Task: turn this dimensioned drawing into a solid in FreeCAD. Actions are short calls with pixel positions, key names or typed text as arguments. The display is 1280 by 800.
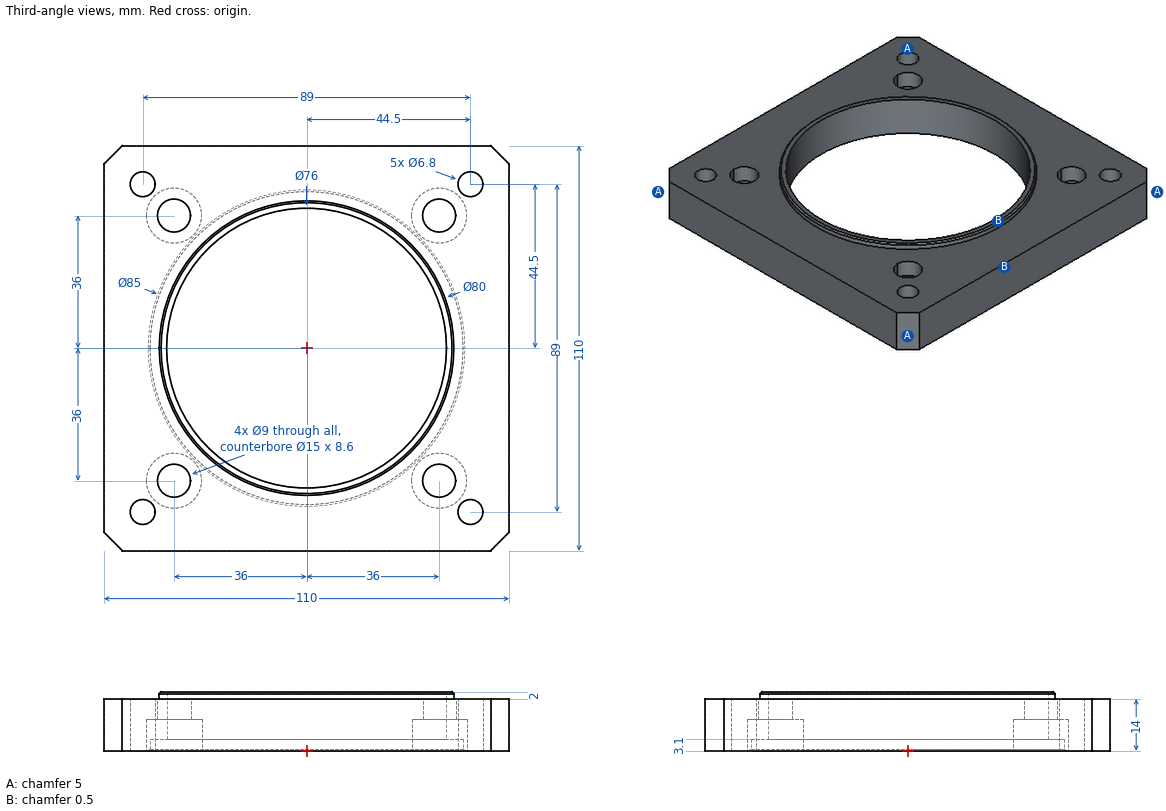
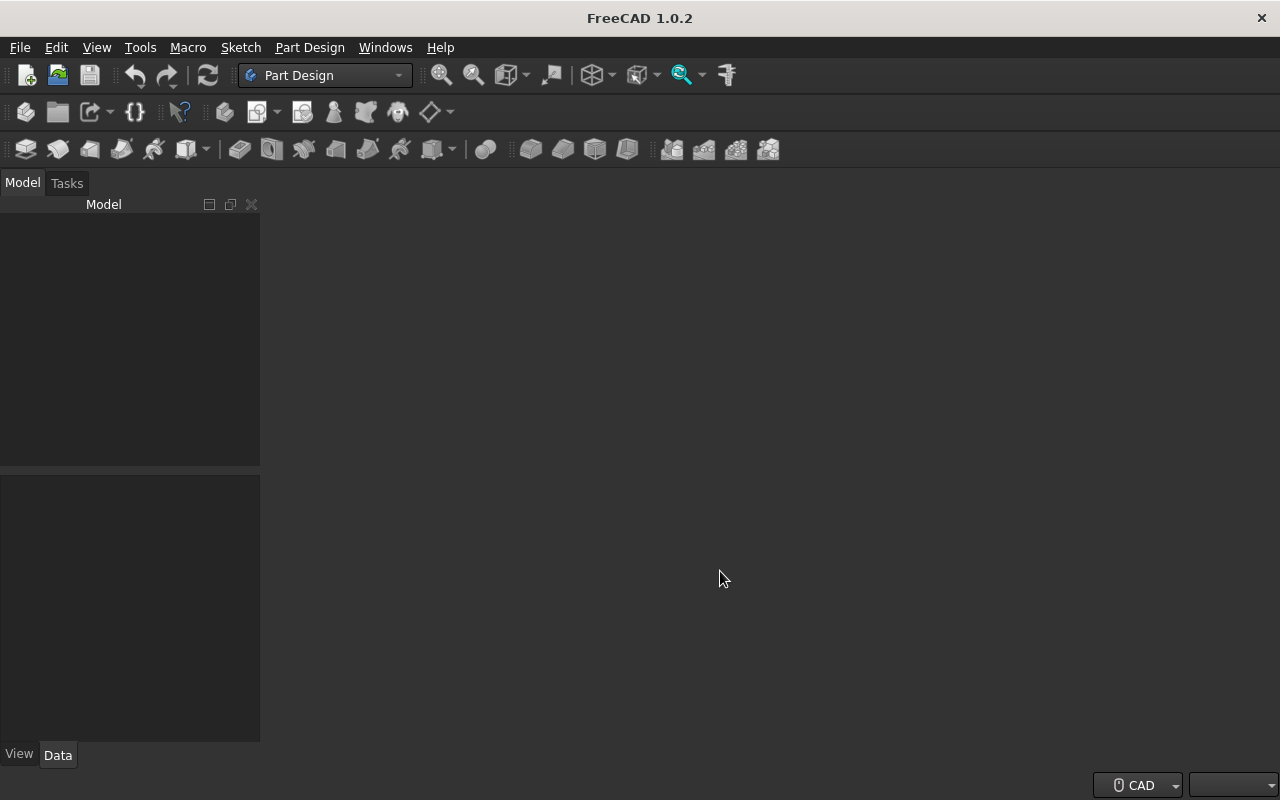
click(26, 76)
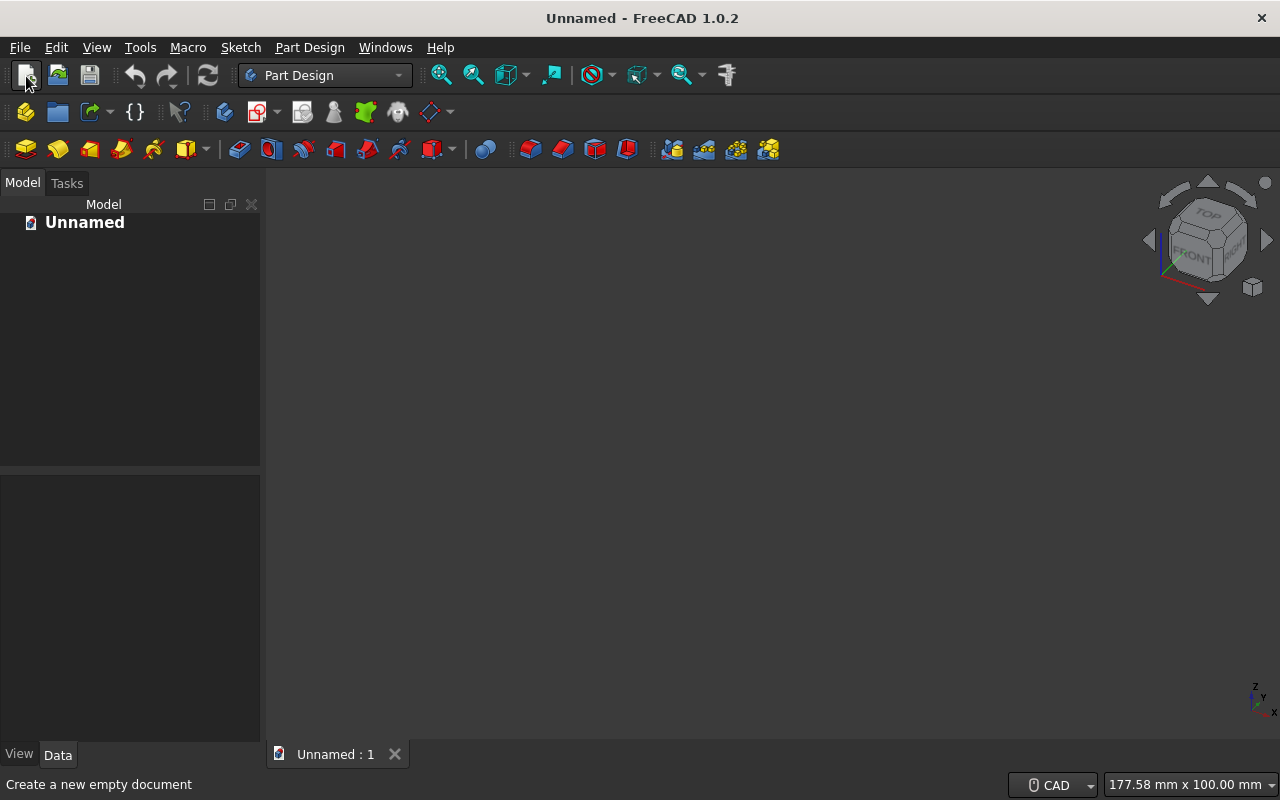
click(258, 112)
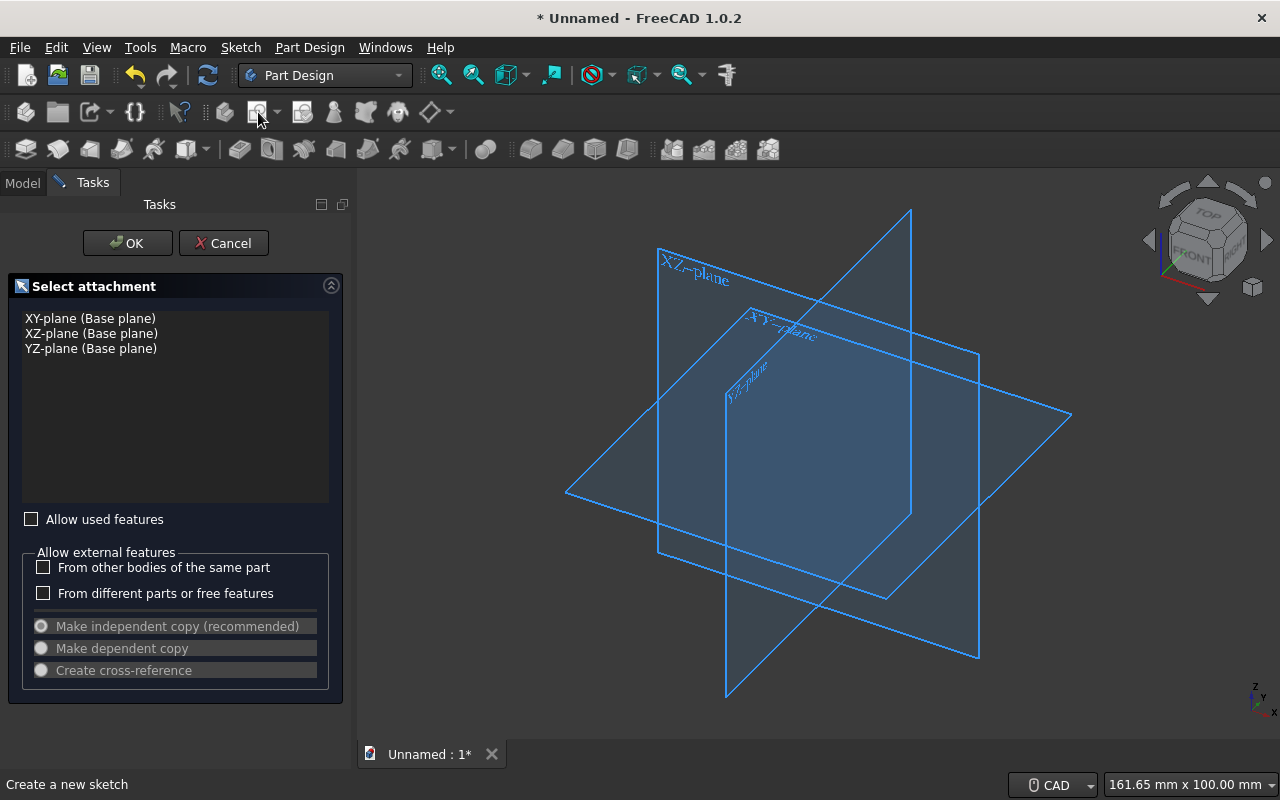
click(82, 318)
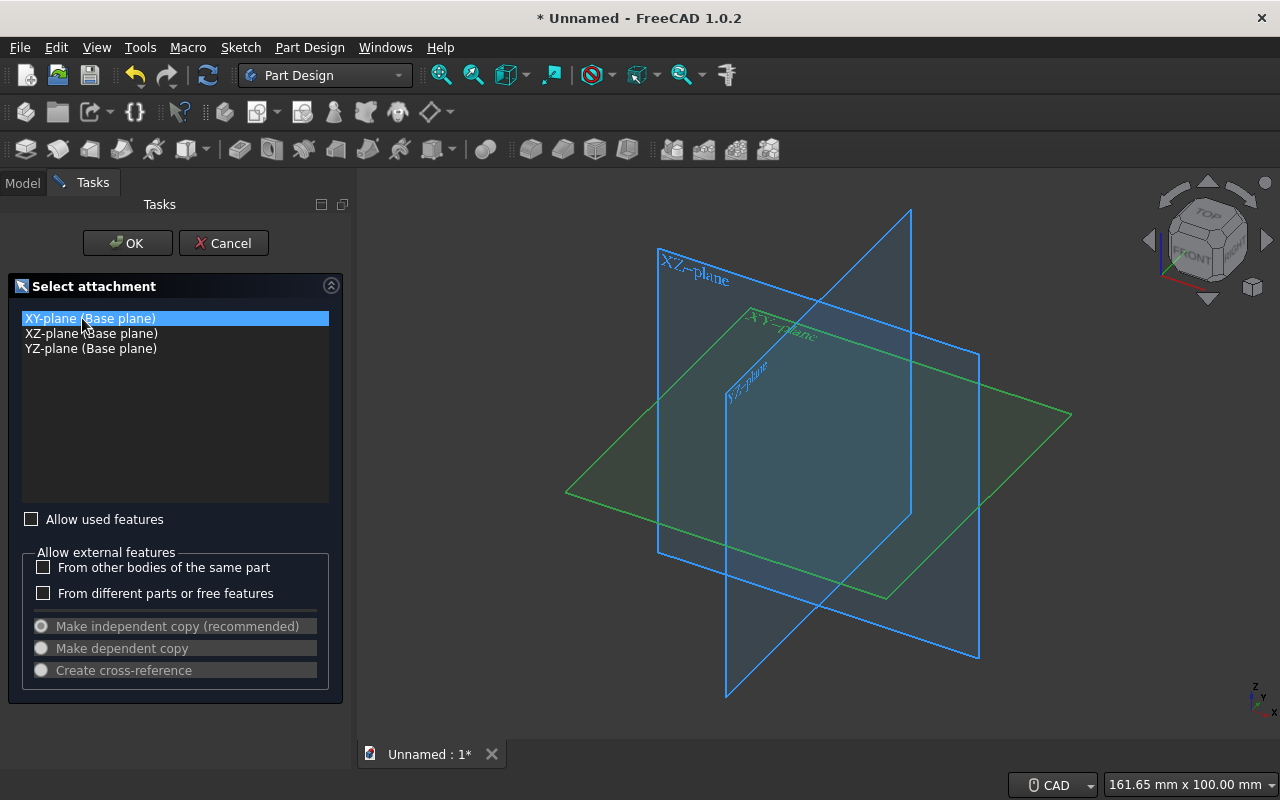
click(128, 243)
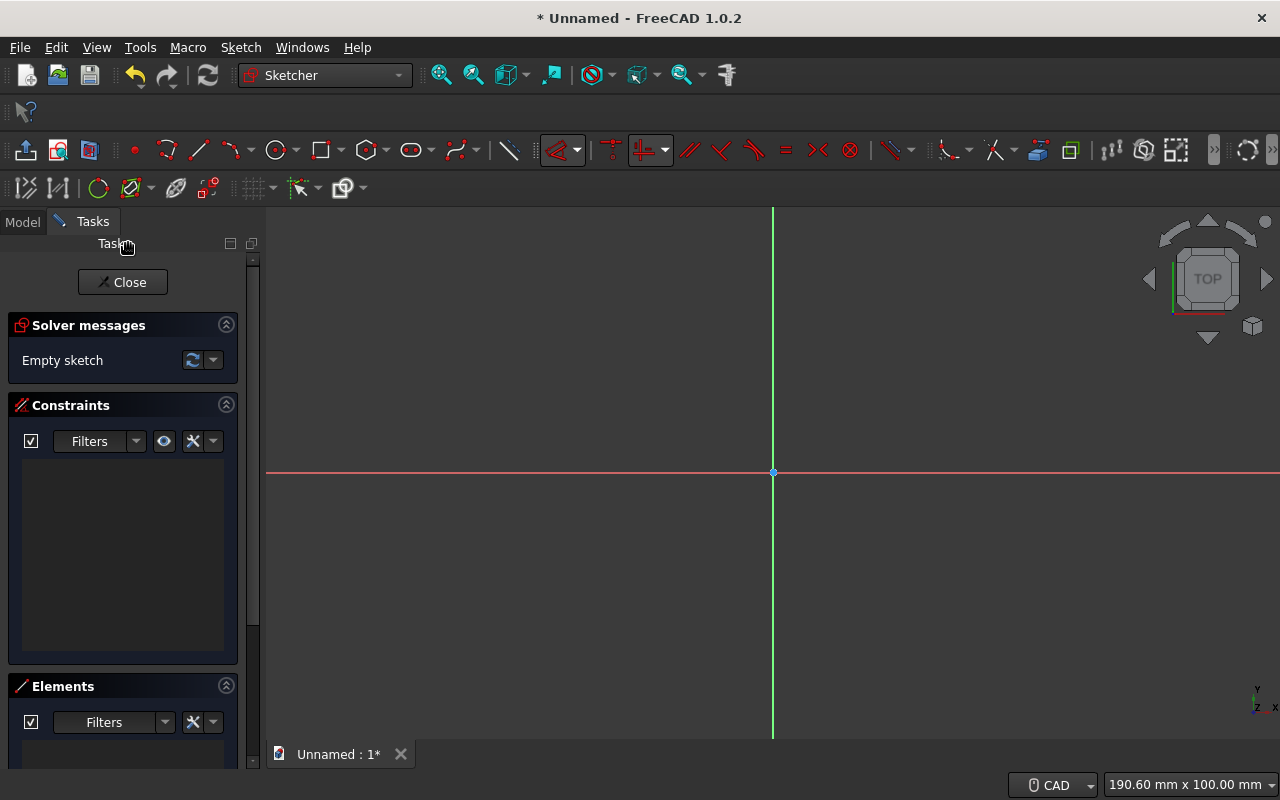
scroll(621, 473, down, 3)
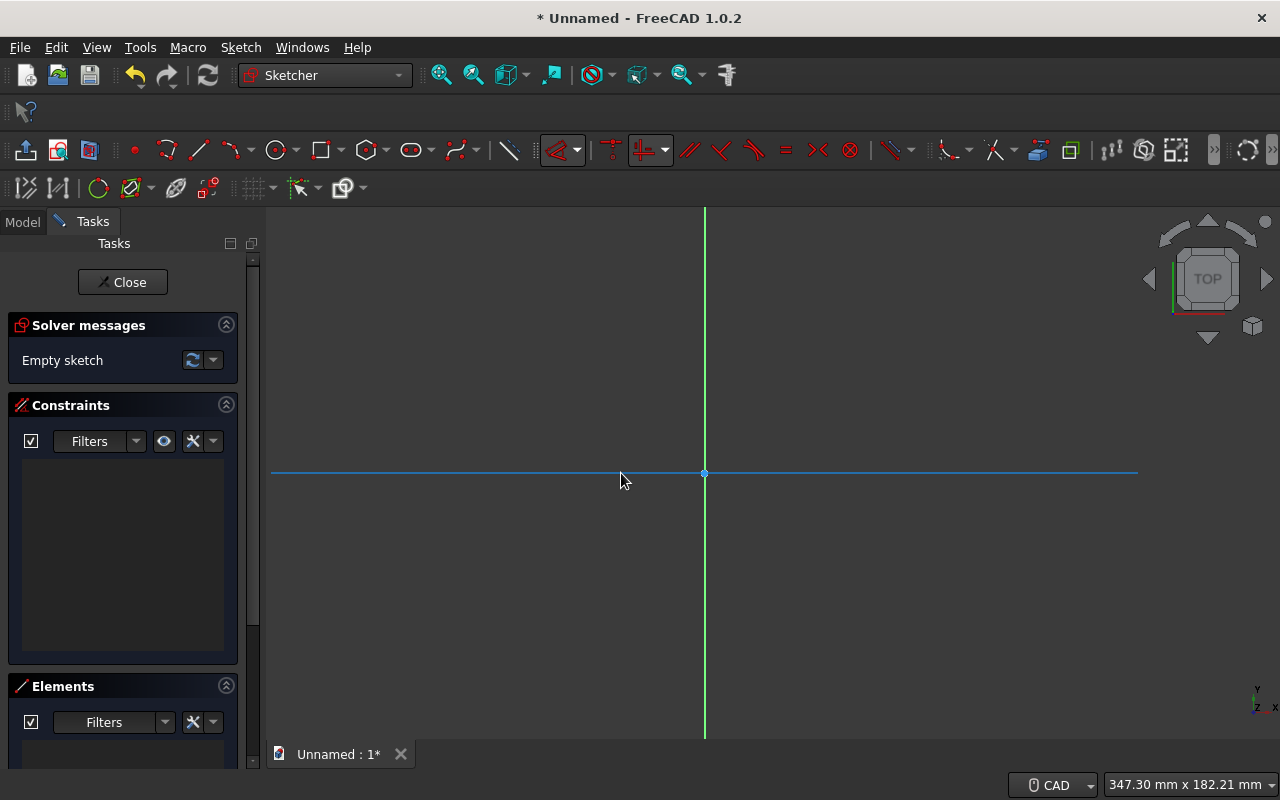
key(g)
key(v)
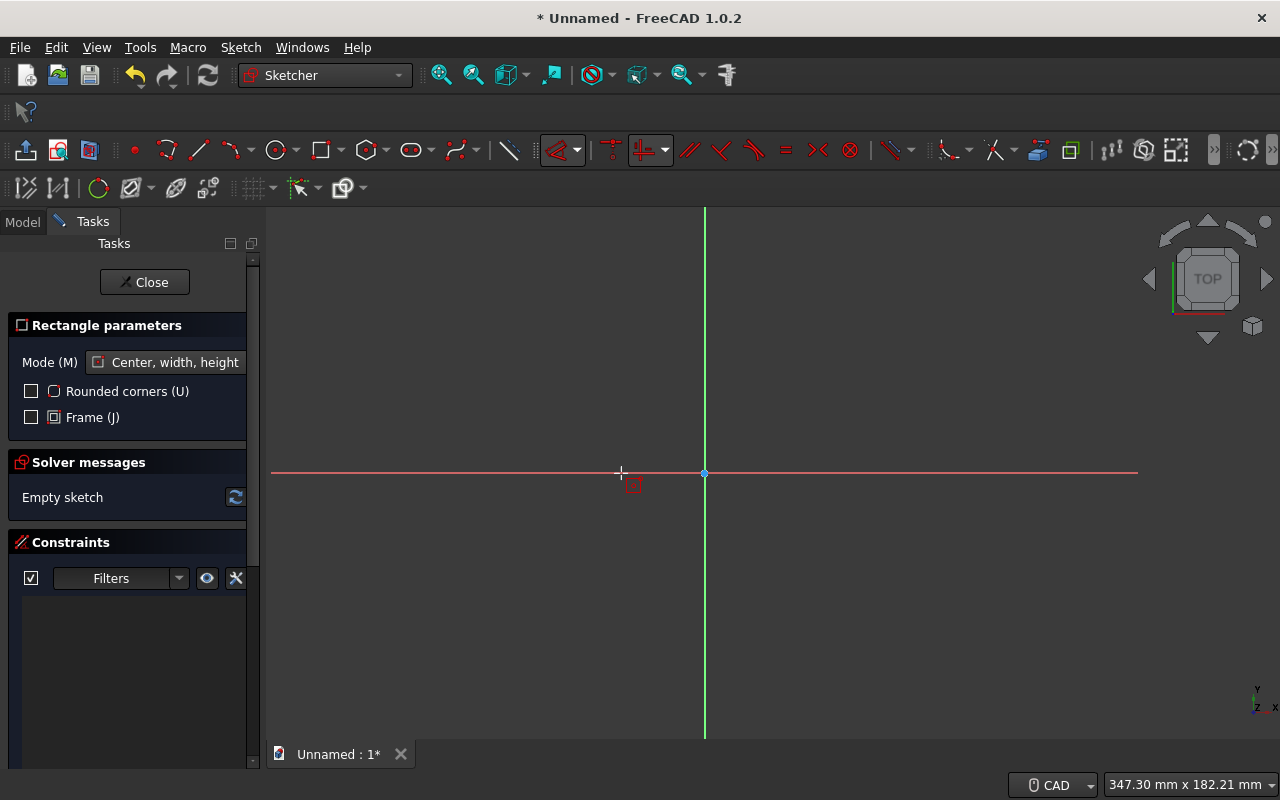
click(705, 473)
click(865, 313)
key(Escape)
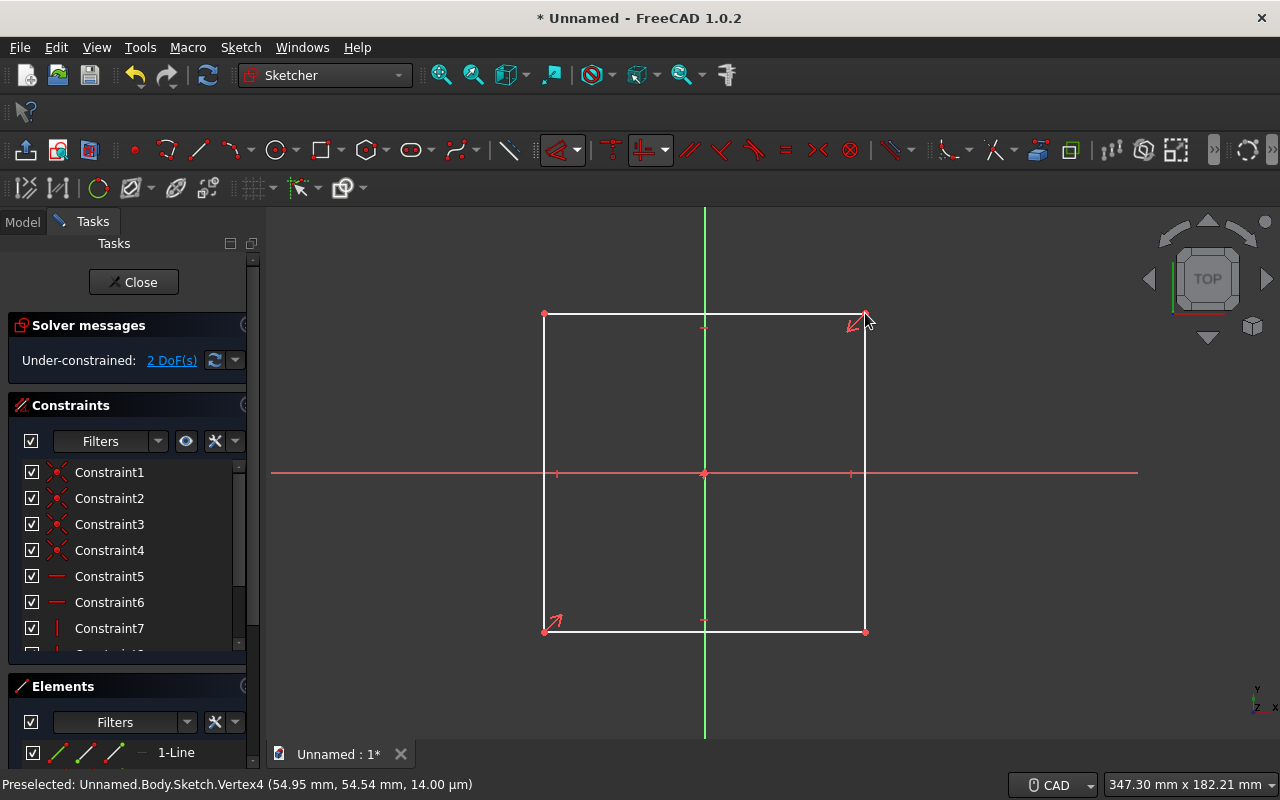
click(640, 632)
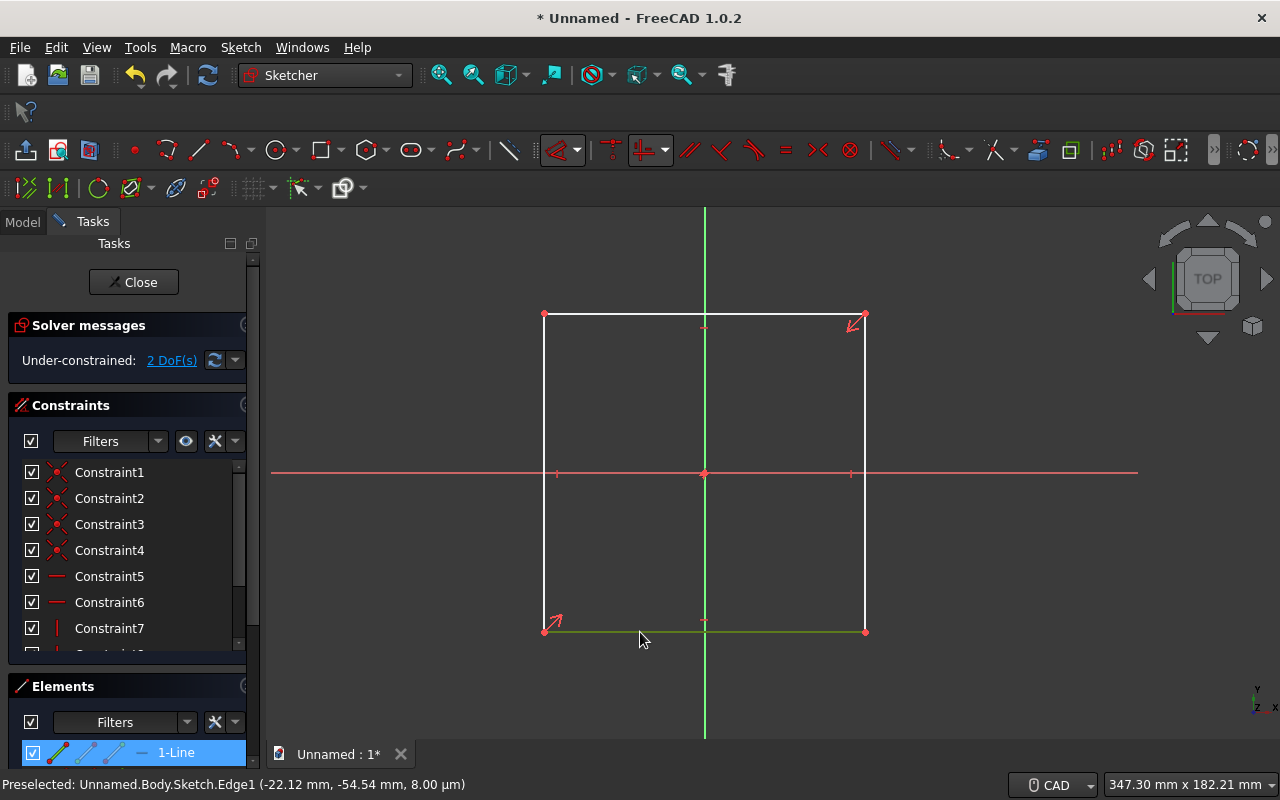
click(580, 150)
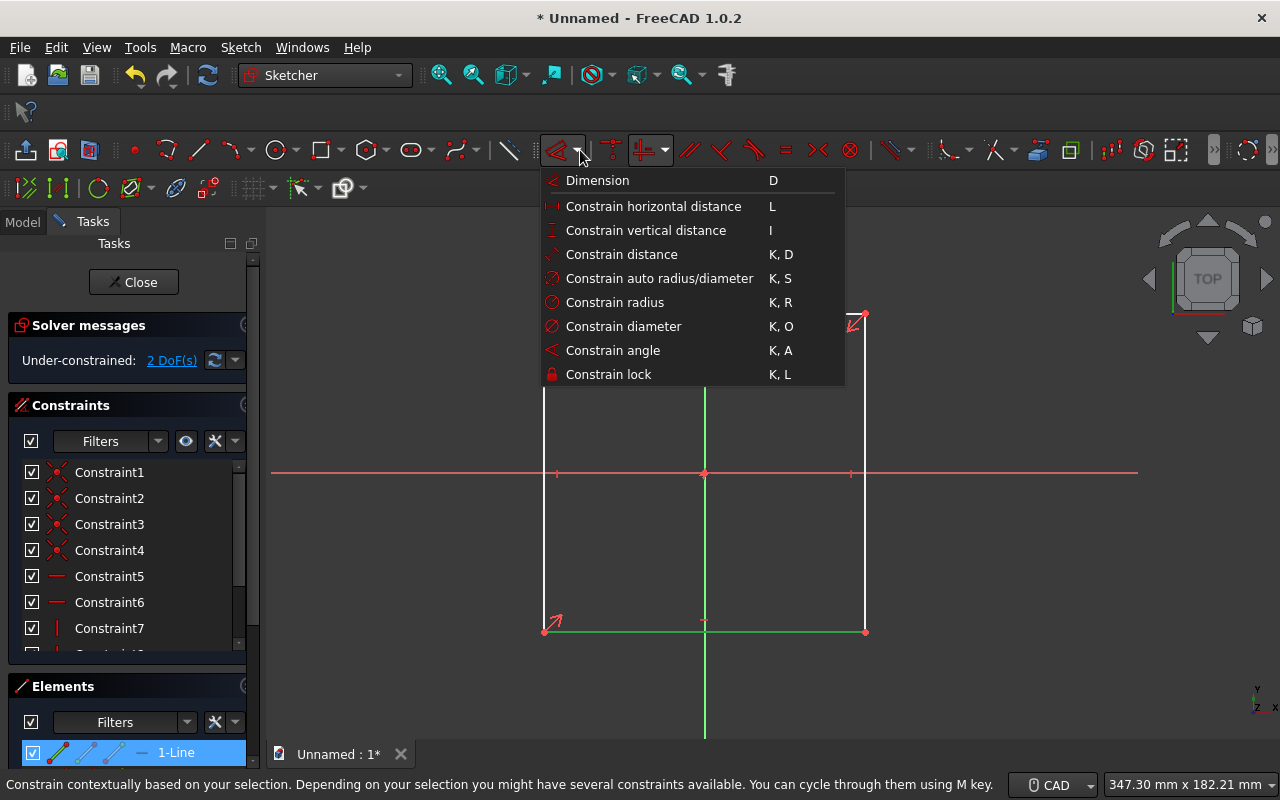
click(693, 206)